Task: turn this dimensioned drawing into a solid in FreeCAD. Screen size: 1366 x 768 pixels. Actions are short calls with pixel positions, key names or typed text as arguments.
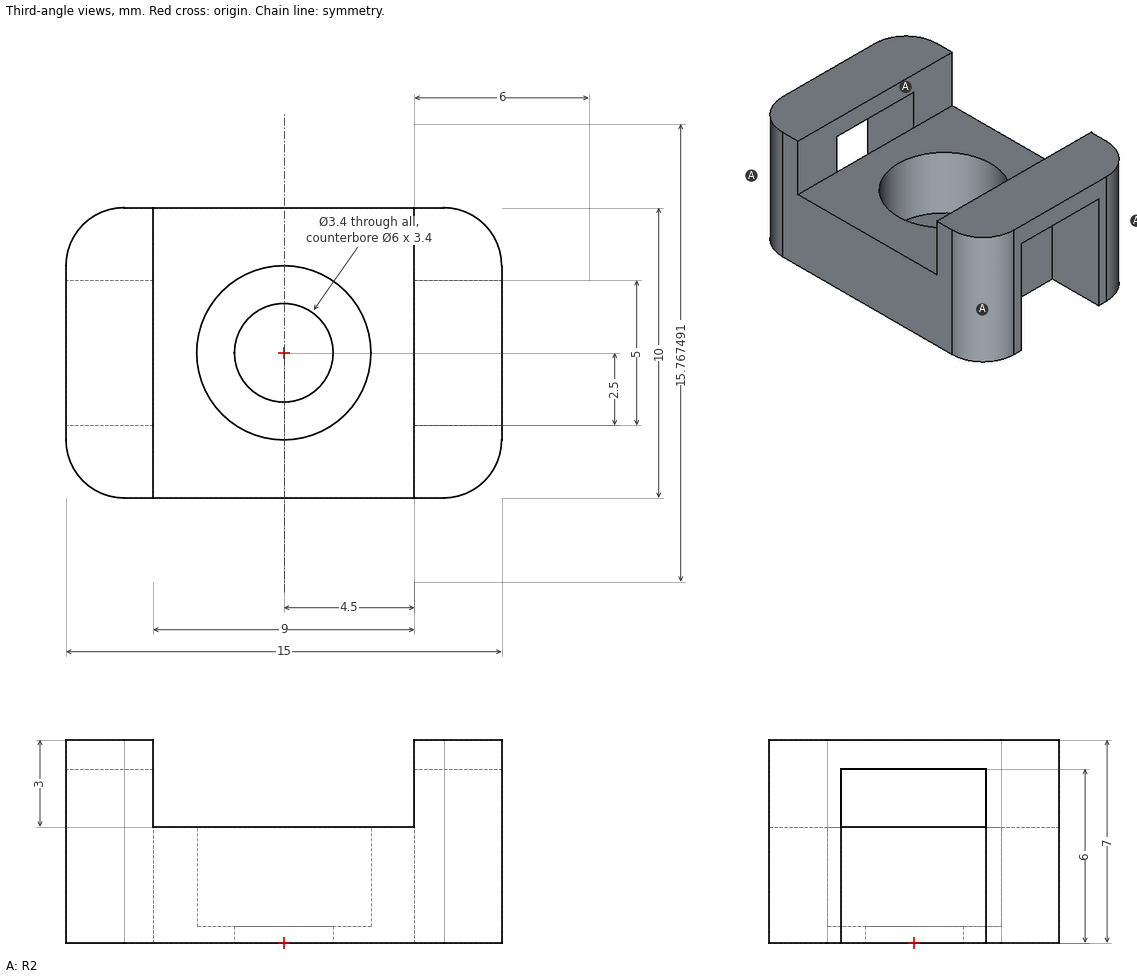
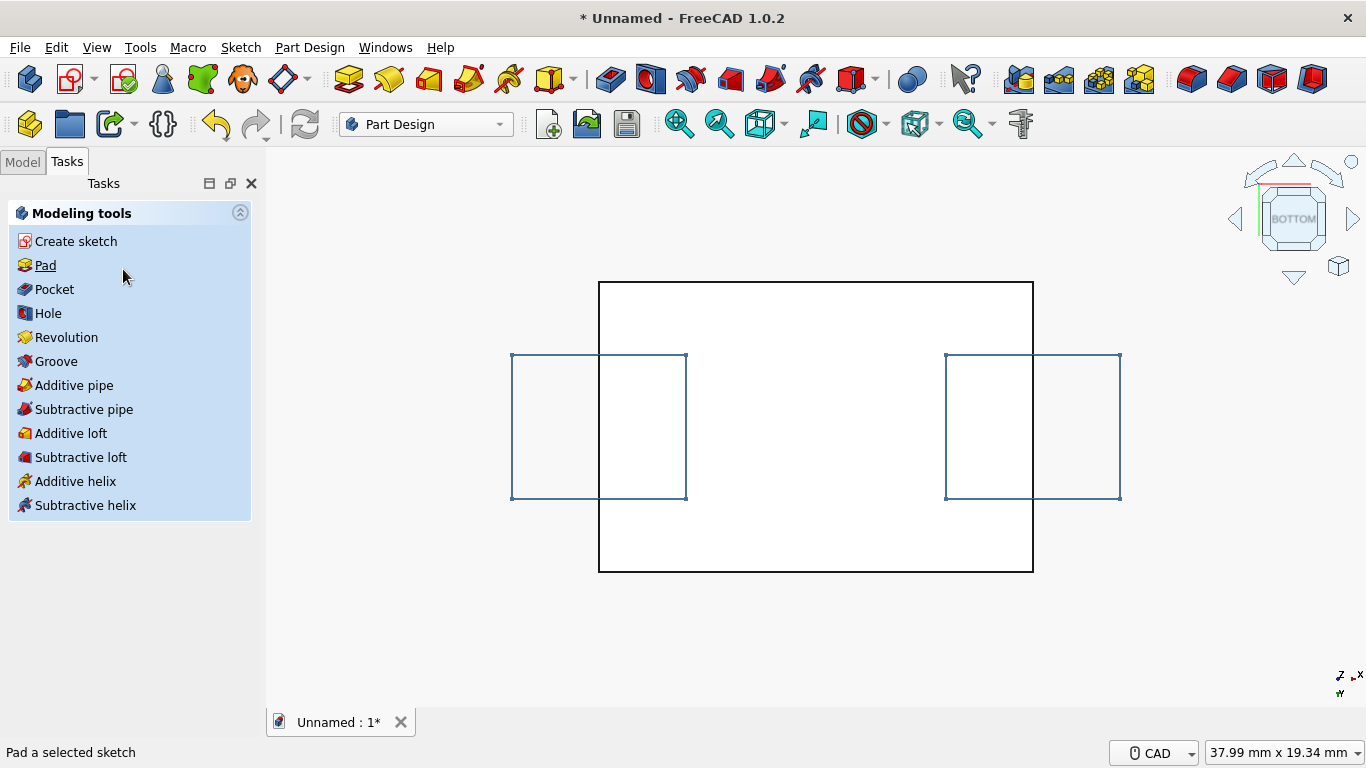
click(612, 80)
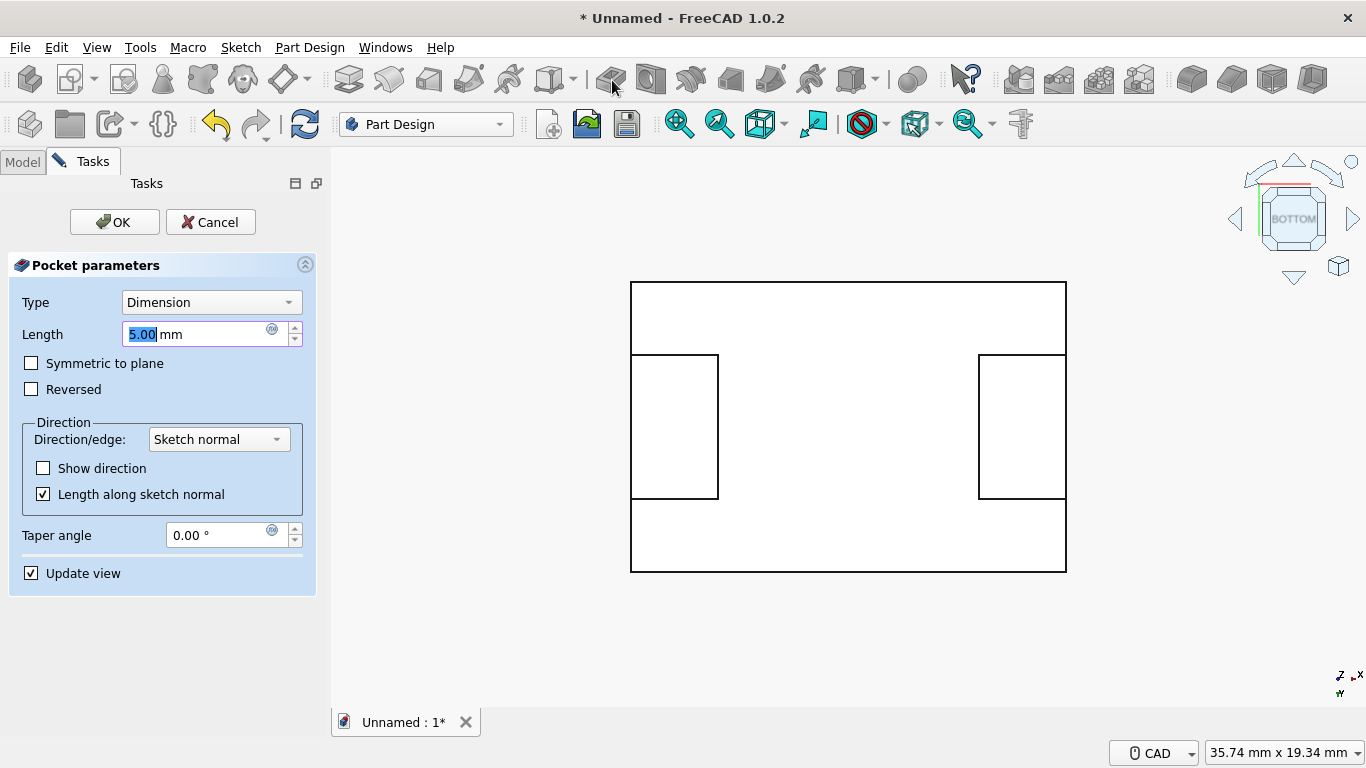
text(6)
key(Tab)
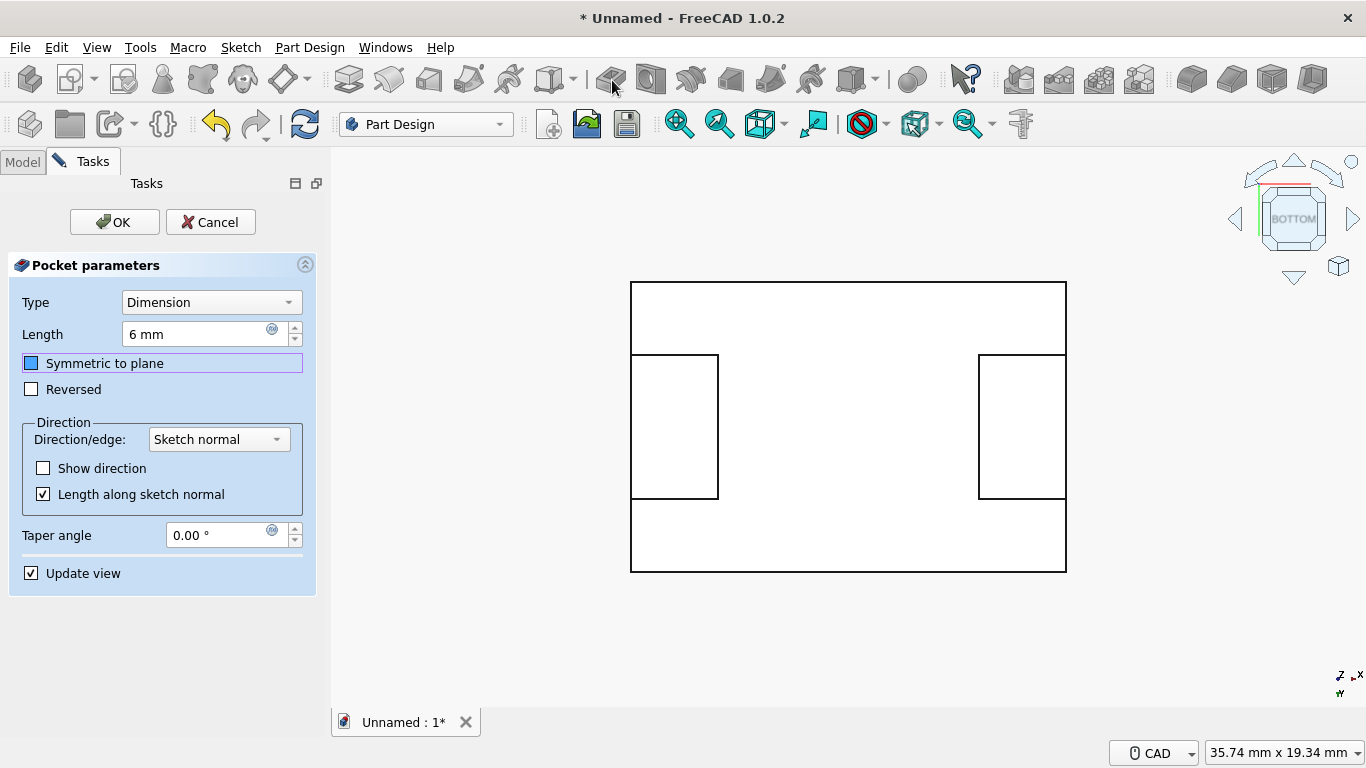
click(115, 222)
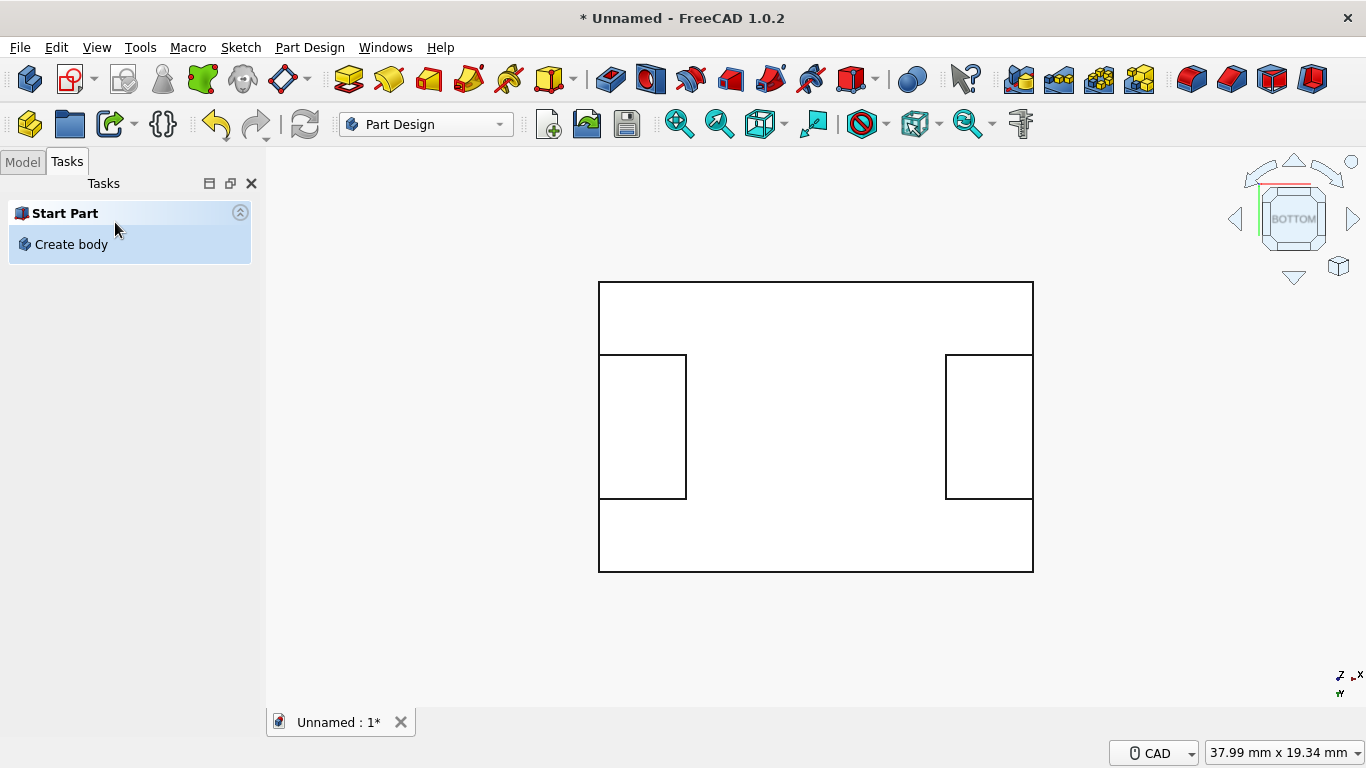
key(0)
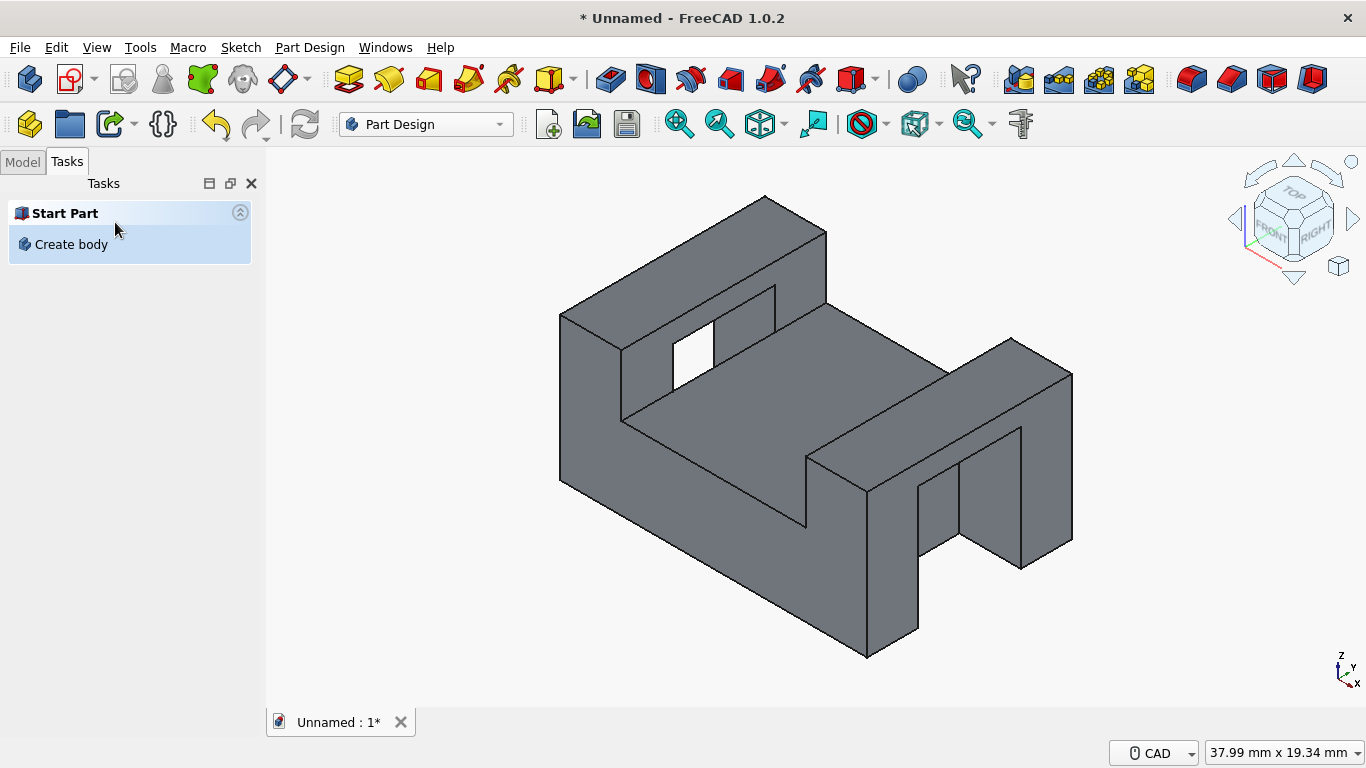
click(816, 414)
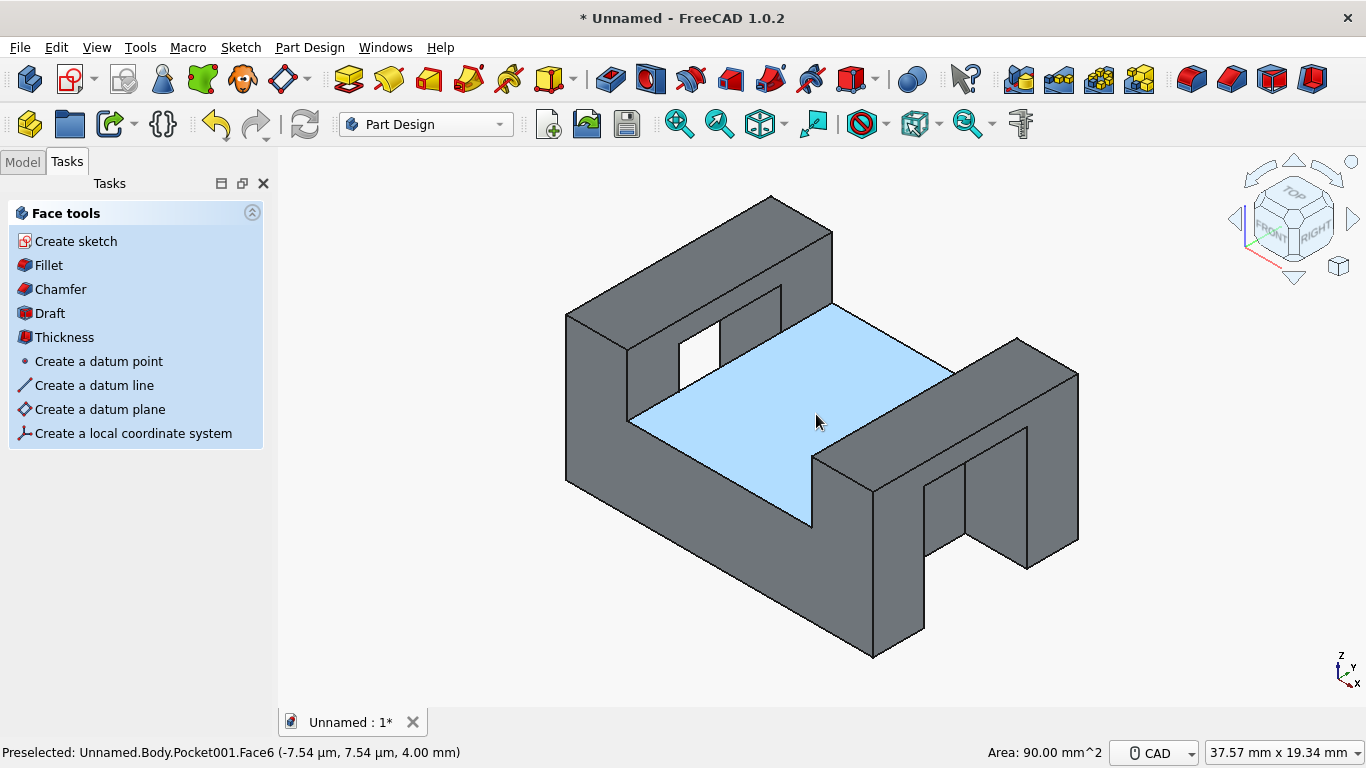
click(70, 80)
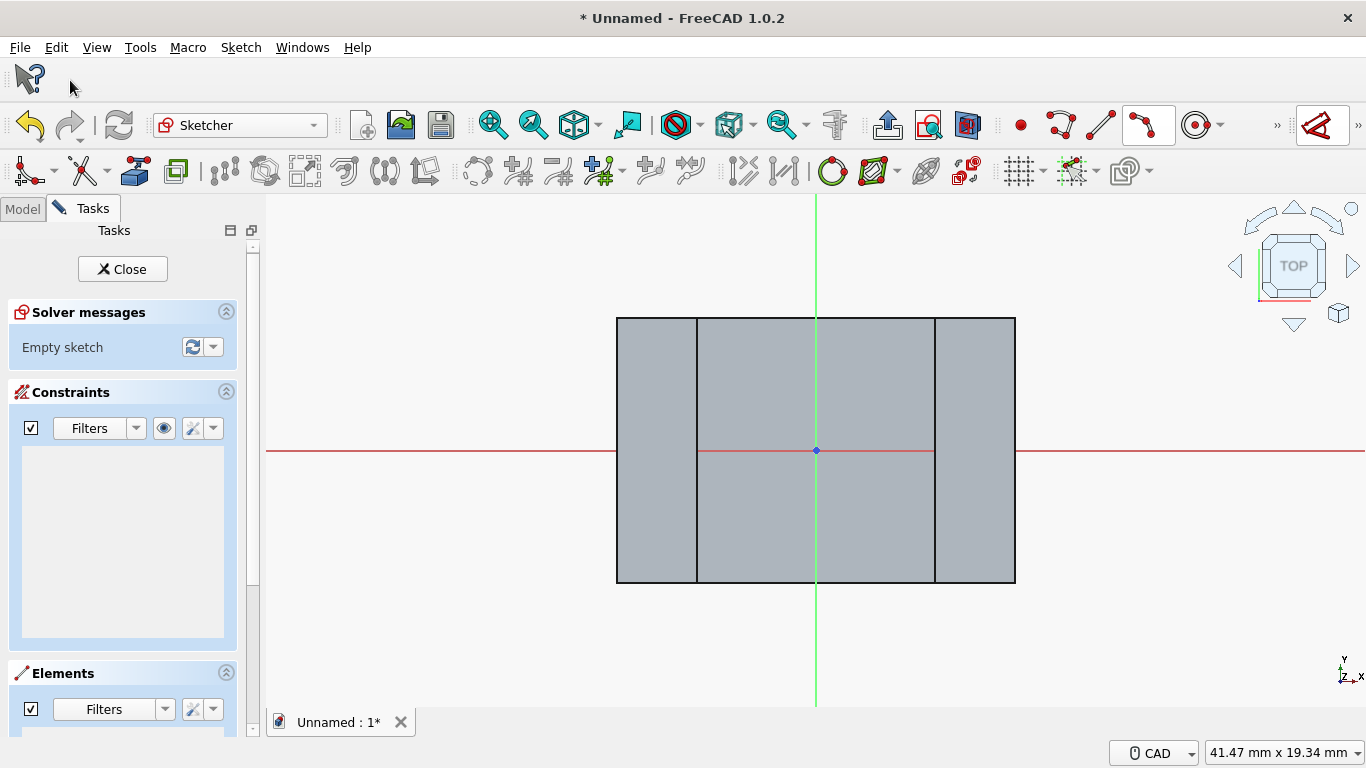
click(968, 126)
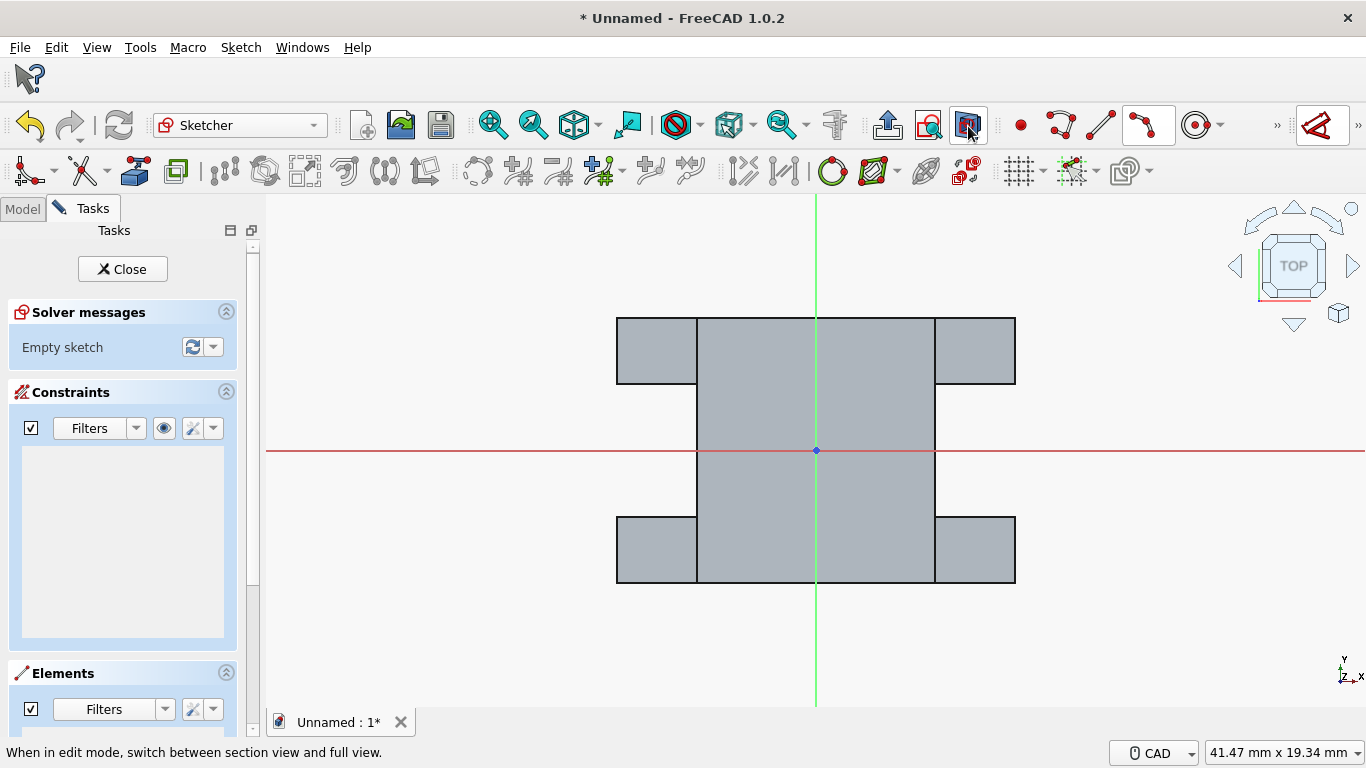
scroll(846, 450, up, 6)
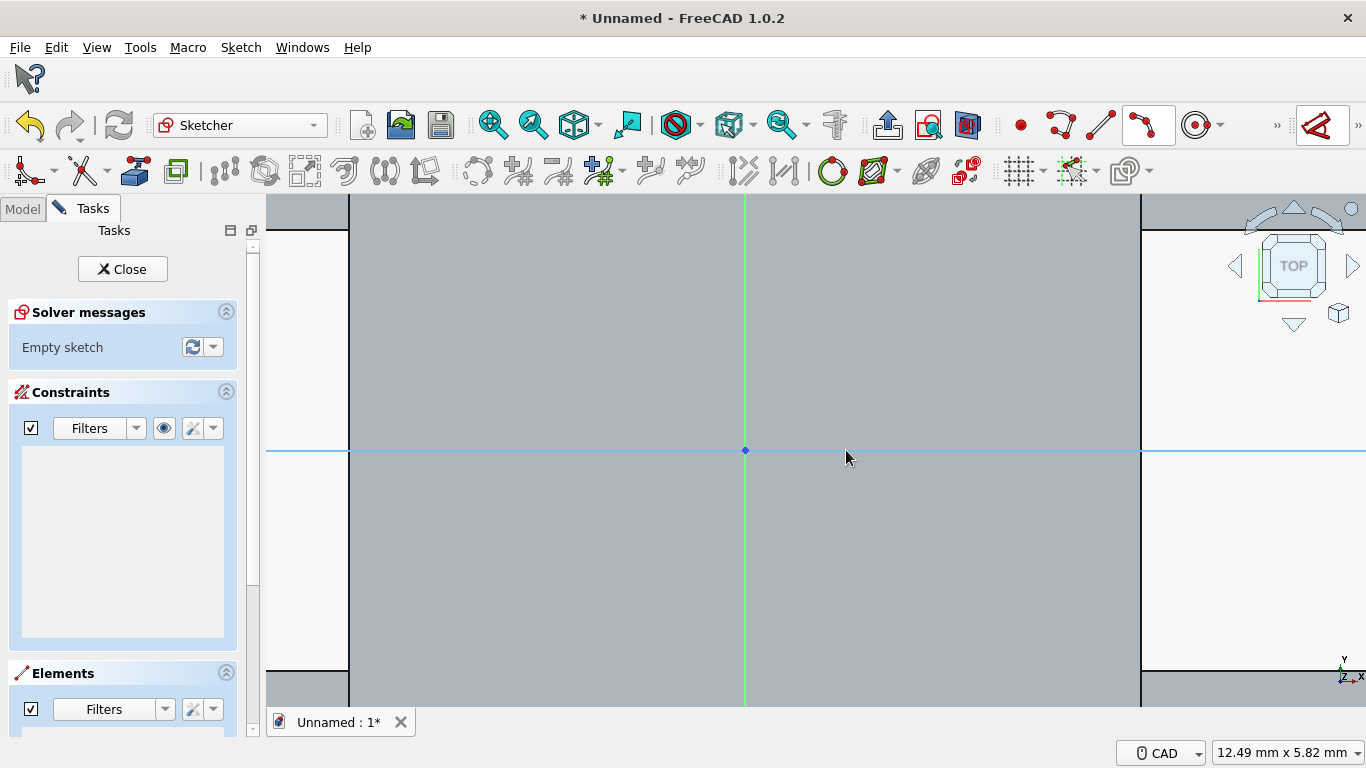
click(1196, 126)